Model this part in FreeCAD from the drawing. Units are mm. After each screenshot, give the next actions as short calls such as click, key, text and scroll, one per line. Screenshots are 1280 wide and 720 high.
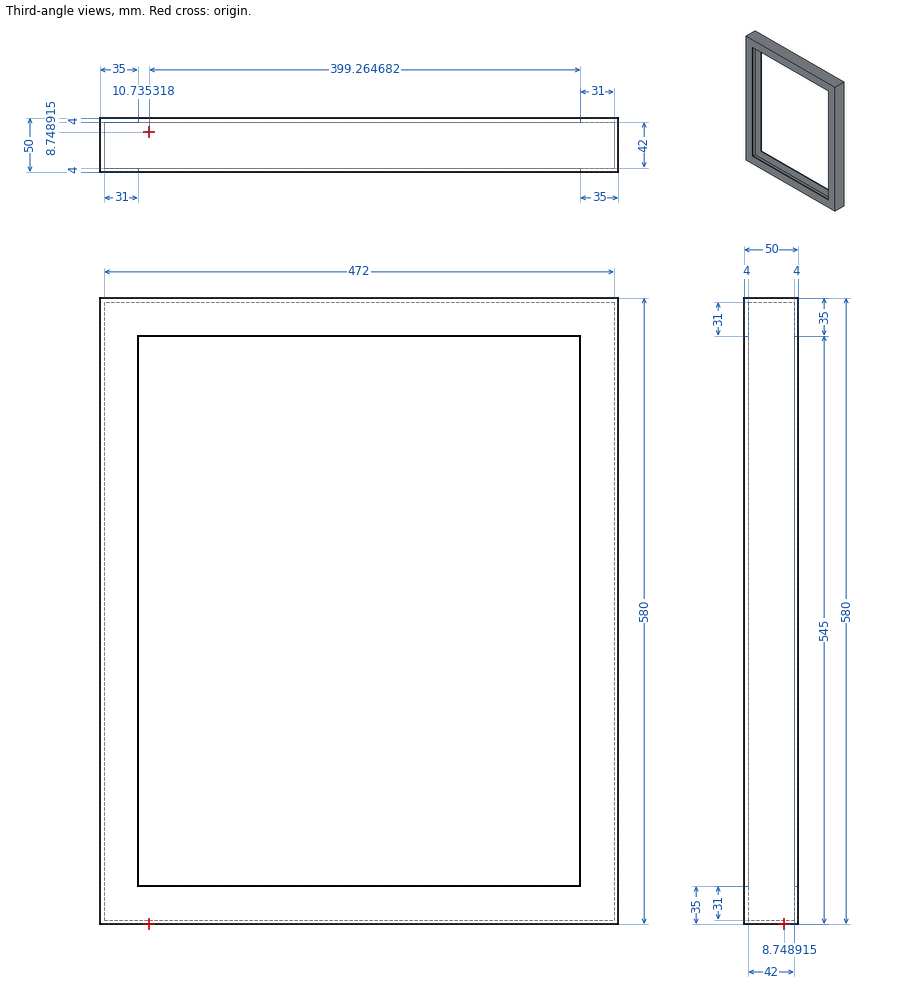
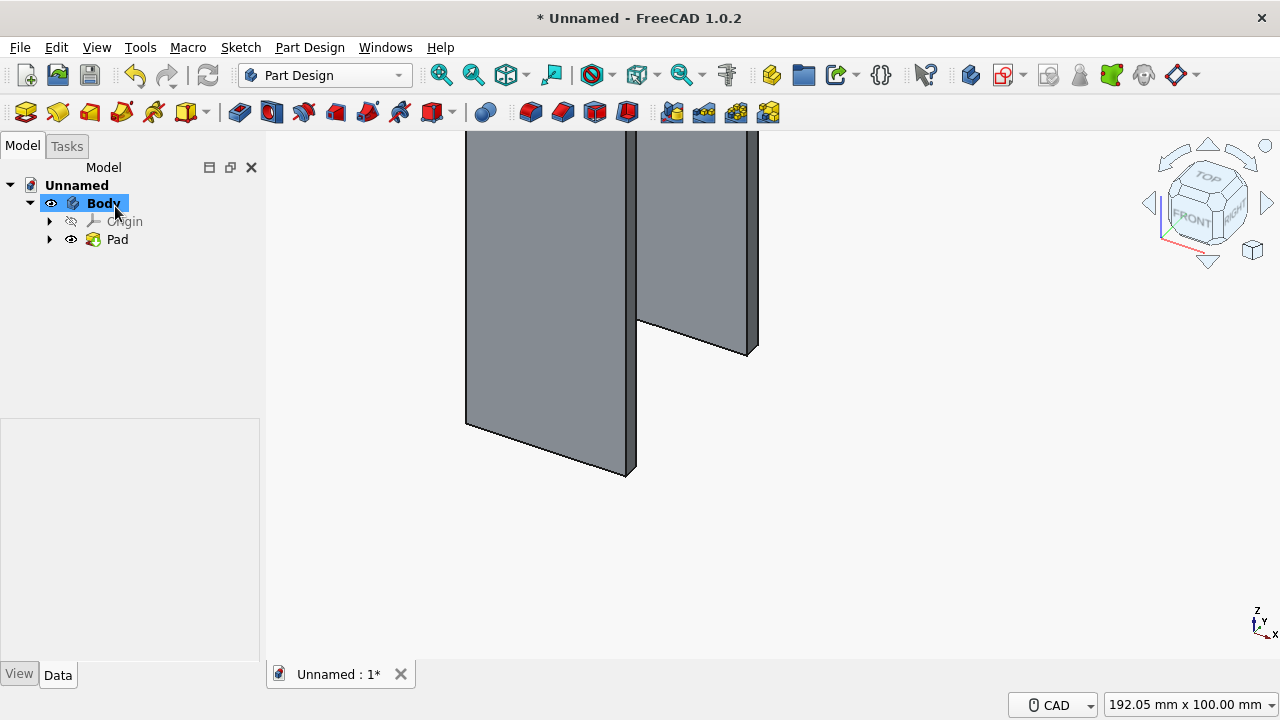
click(442, 76)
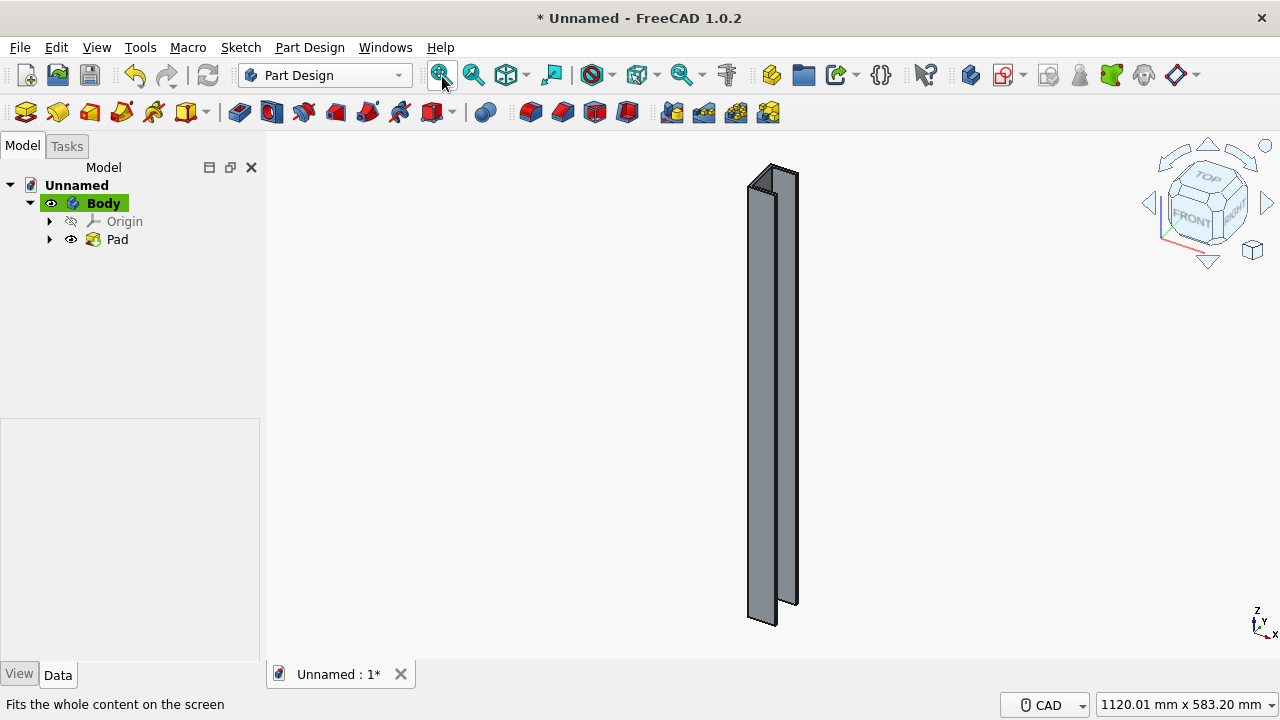
key(0)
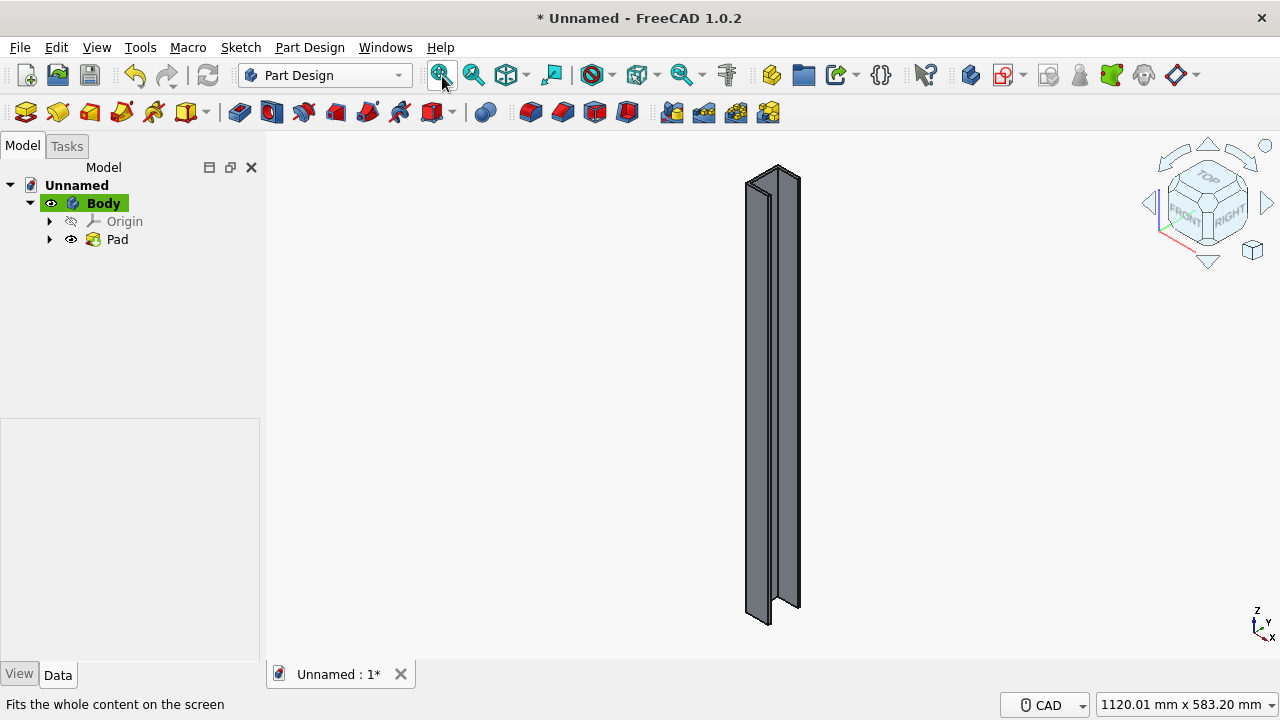
key(3)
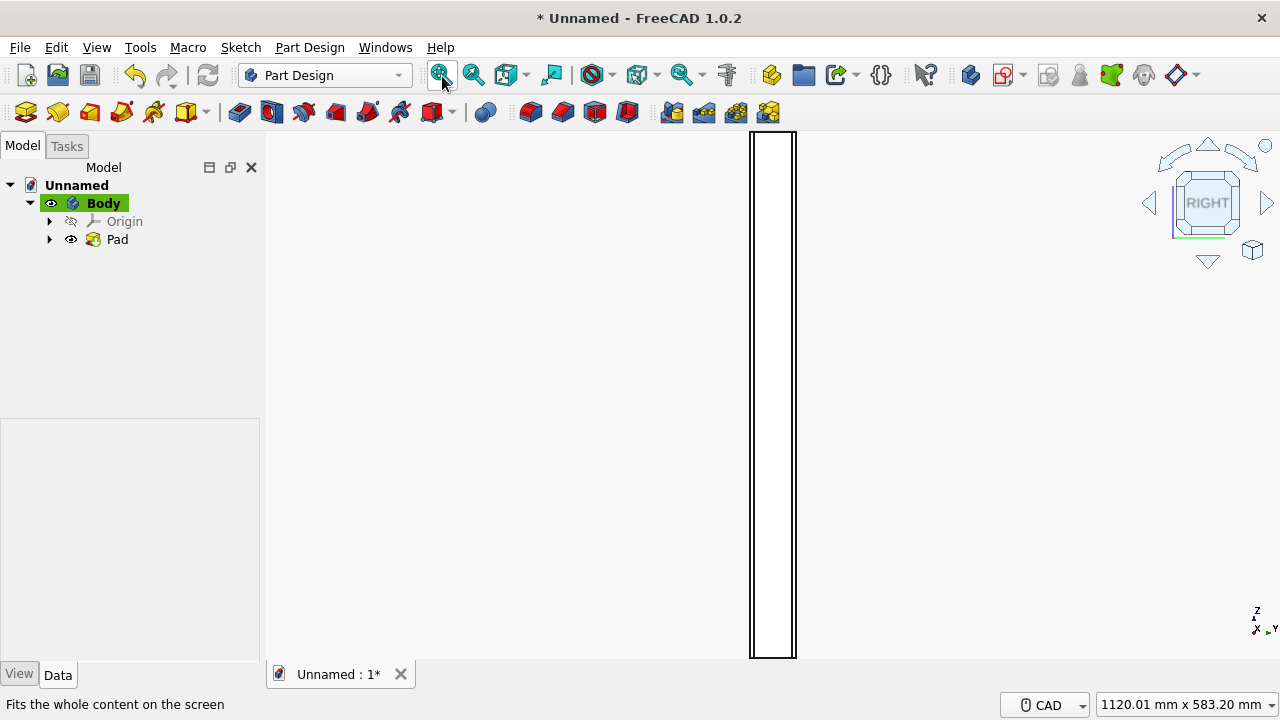
click(773, 169)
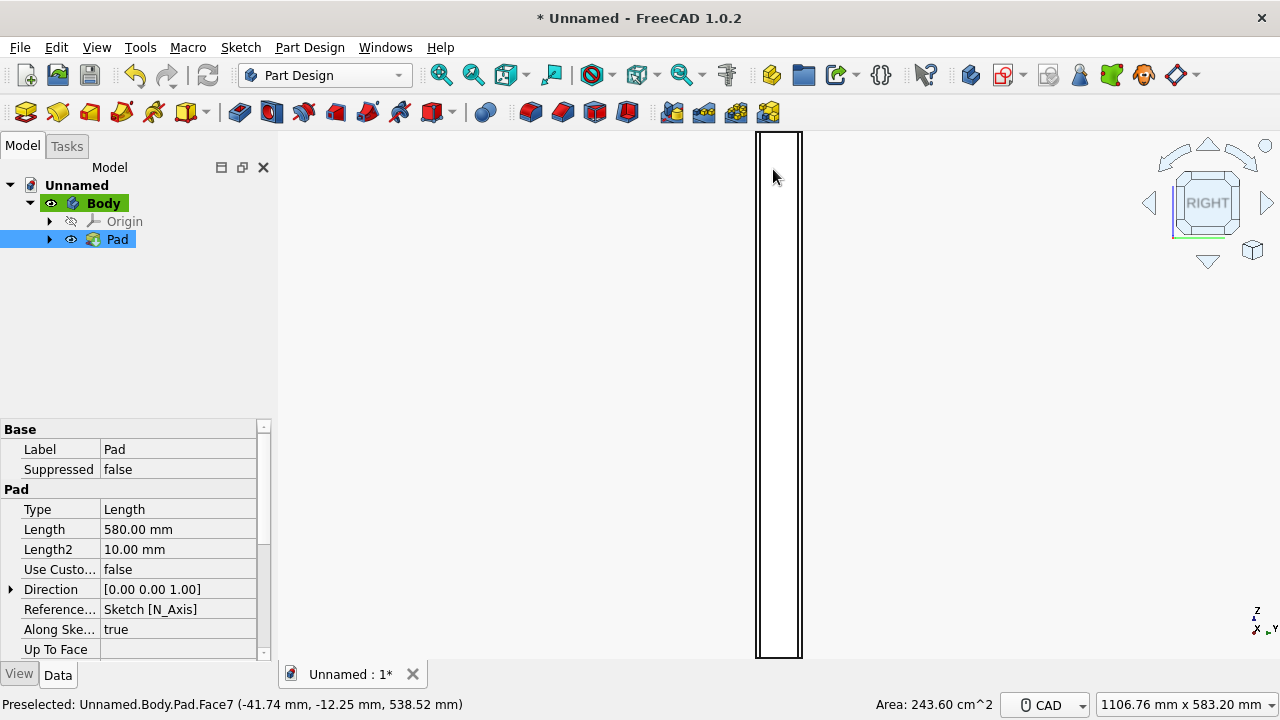
click(1004, 76)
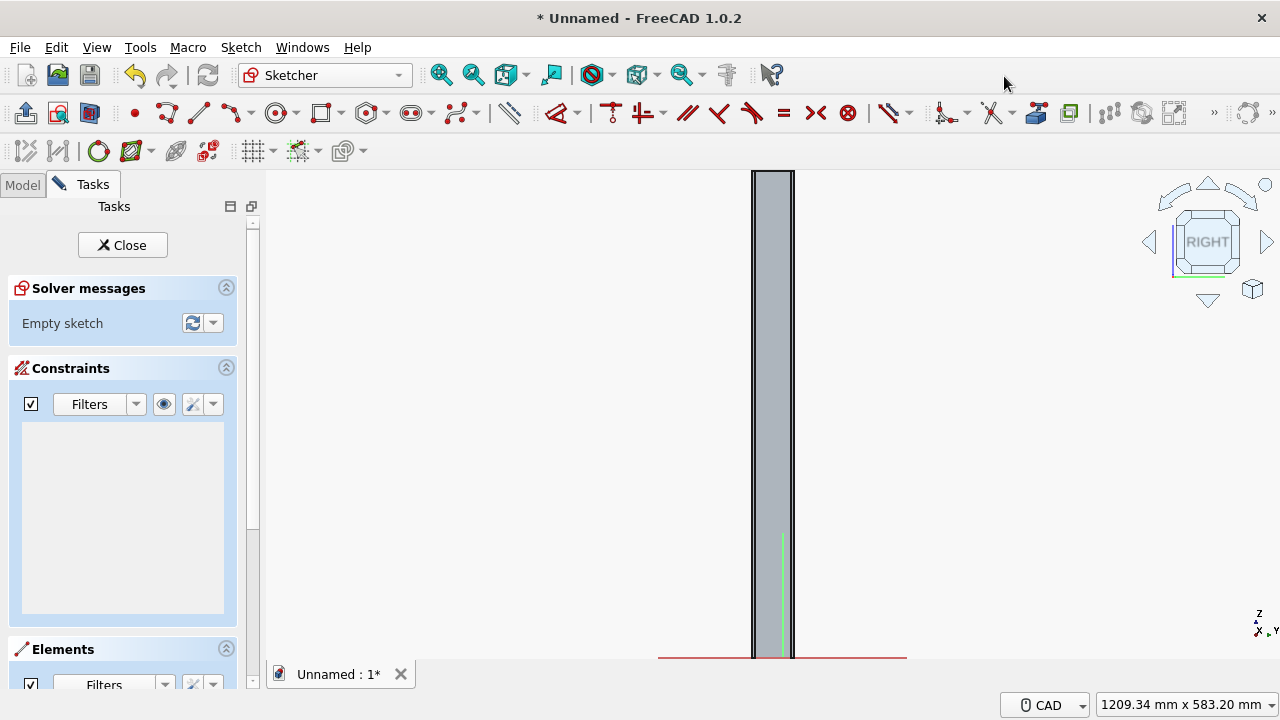
click(90, 114)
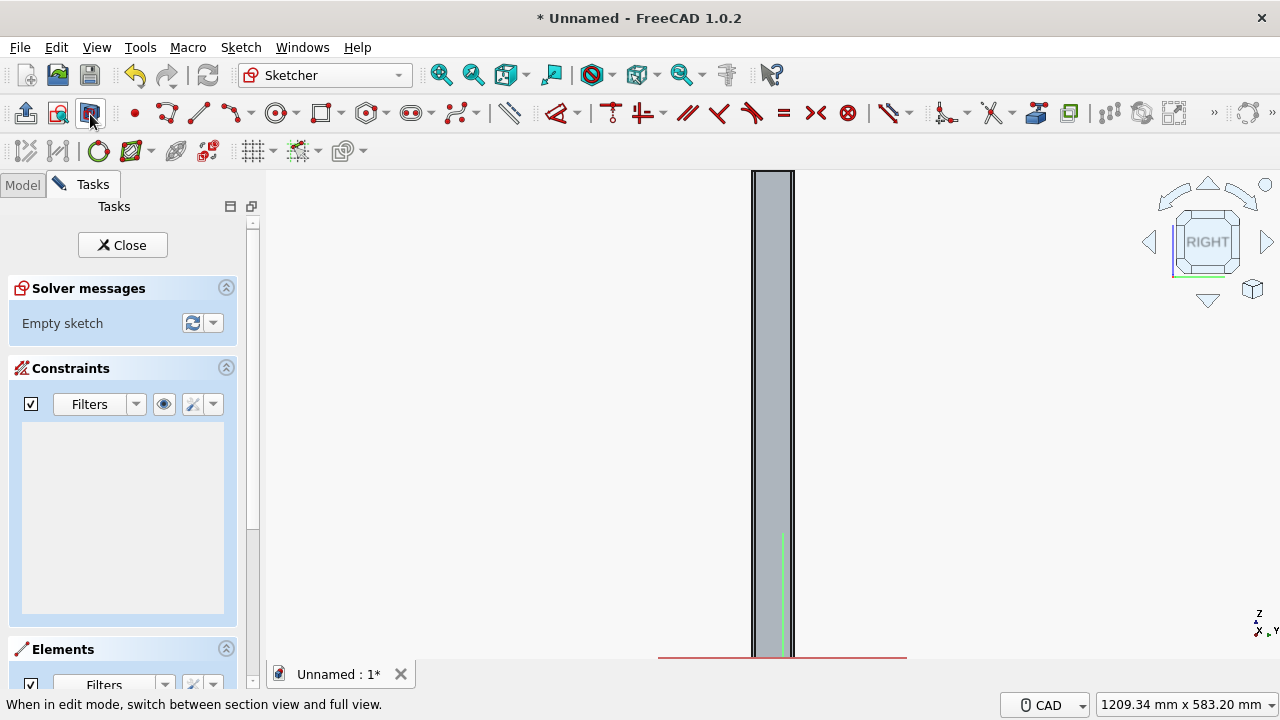
scroll(565, 414, down, 2)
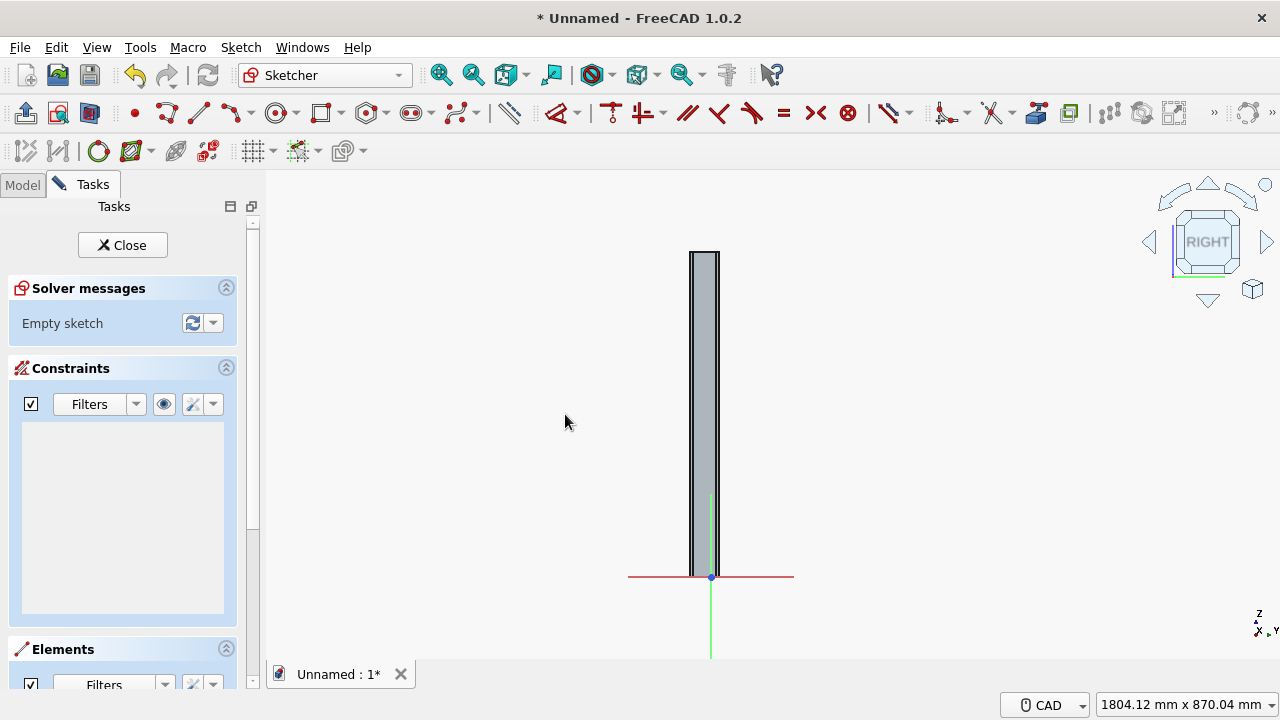
click(168, 114)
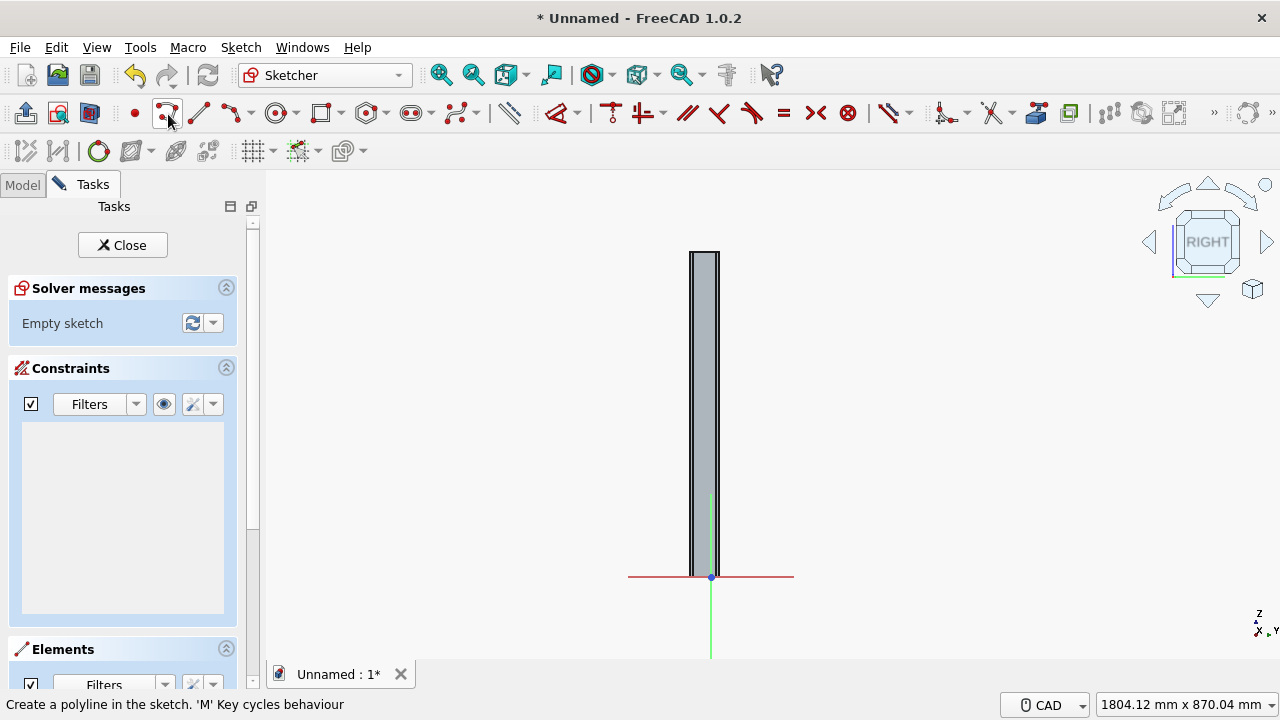
scroll(716, 271, up, 6)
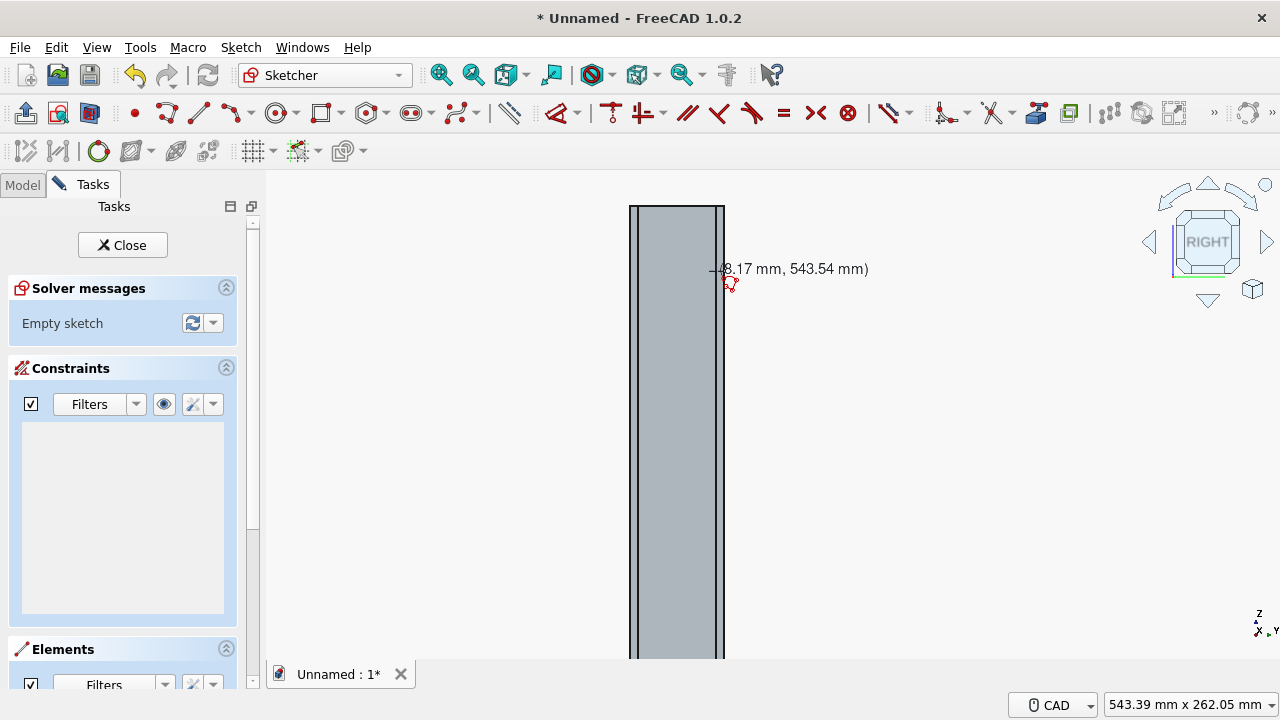
click(716, 271)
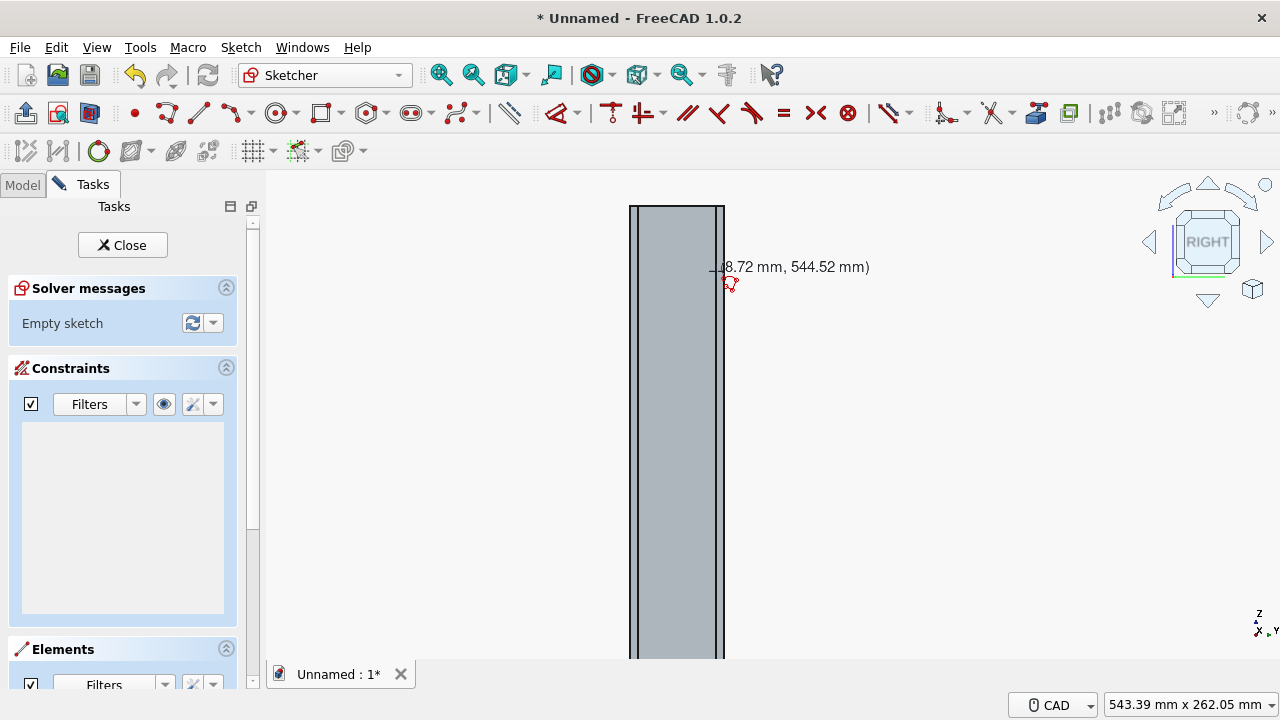
scroll(724, 271, up, 4)